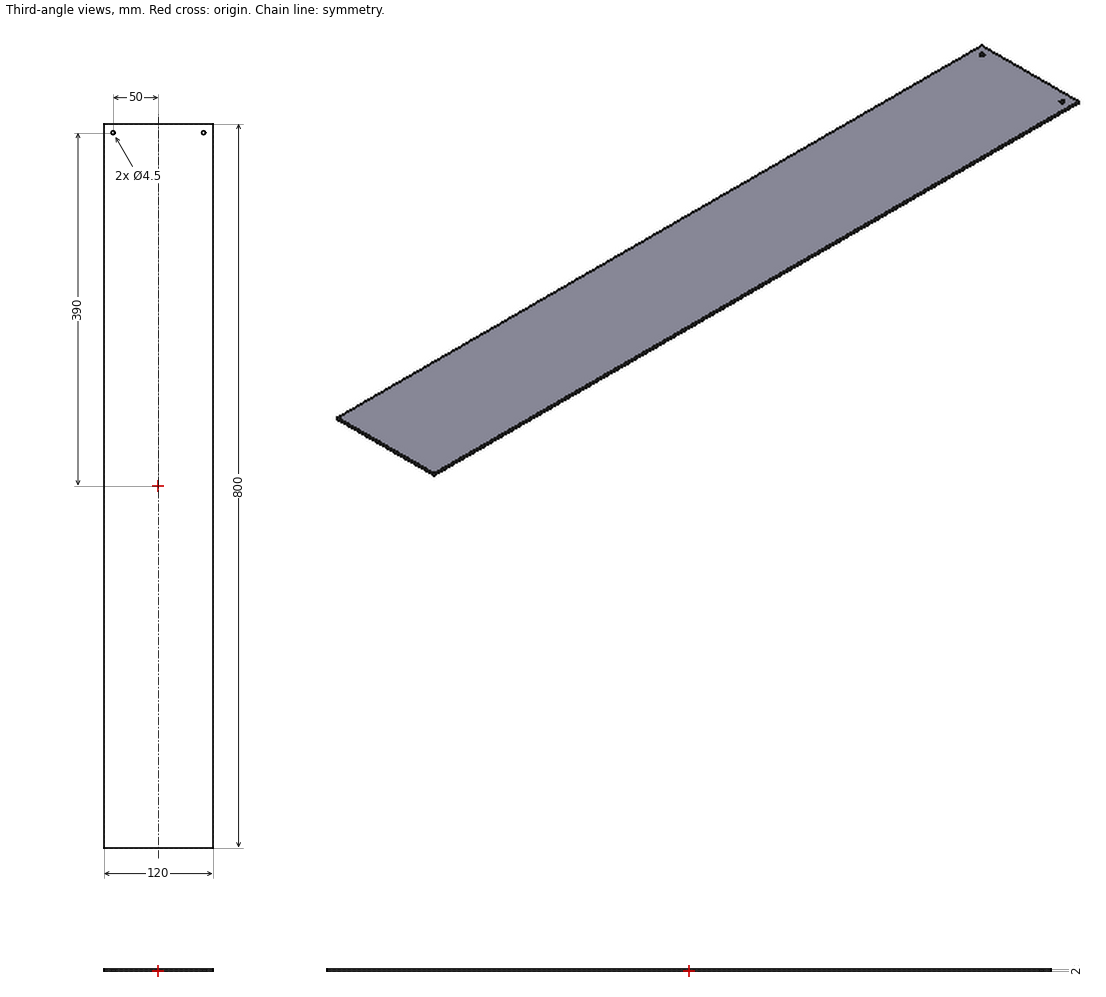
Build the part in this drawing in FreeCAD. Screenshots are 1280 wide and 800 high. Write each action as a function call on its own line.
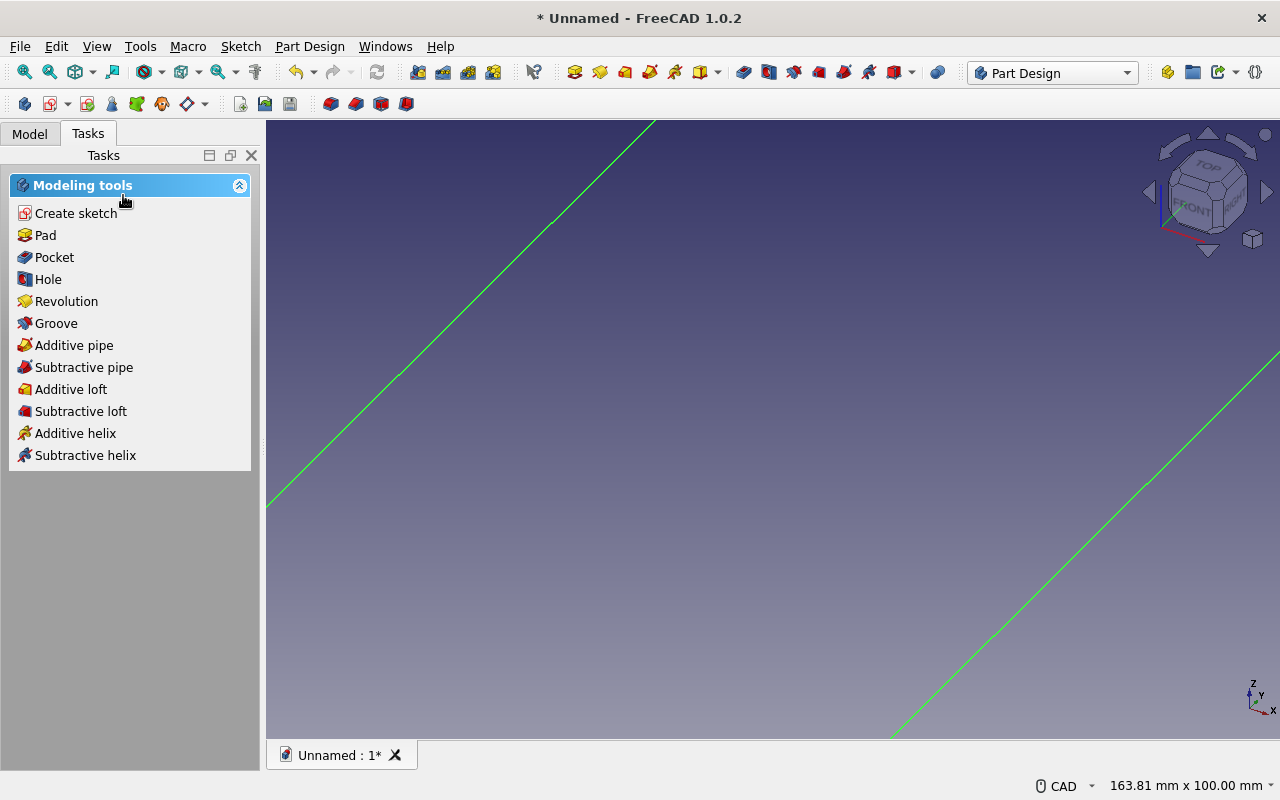
click(575, 72)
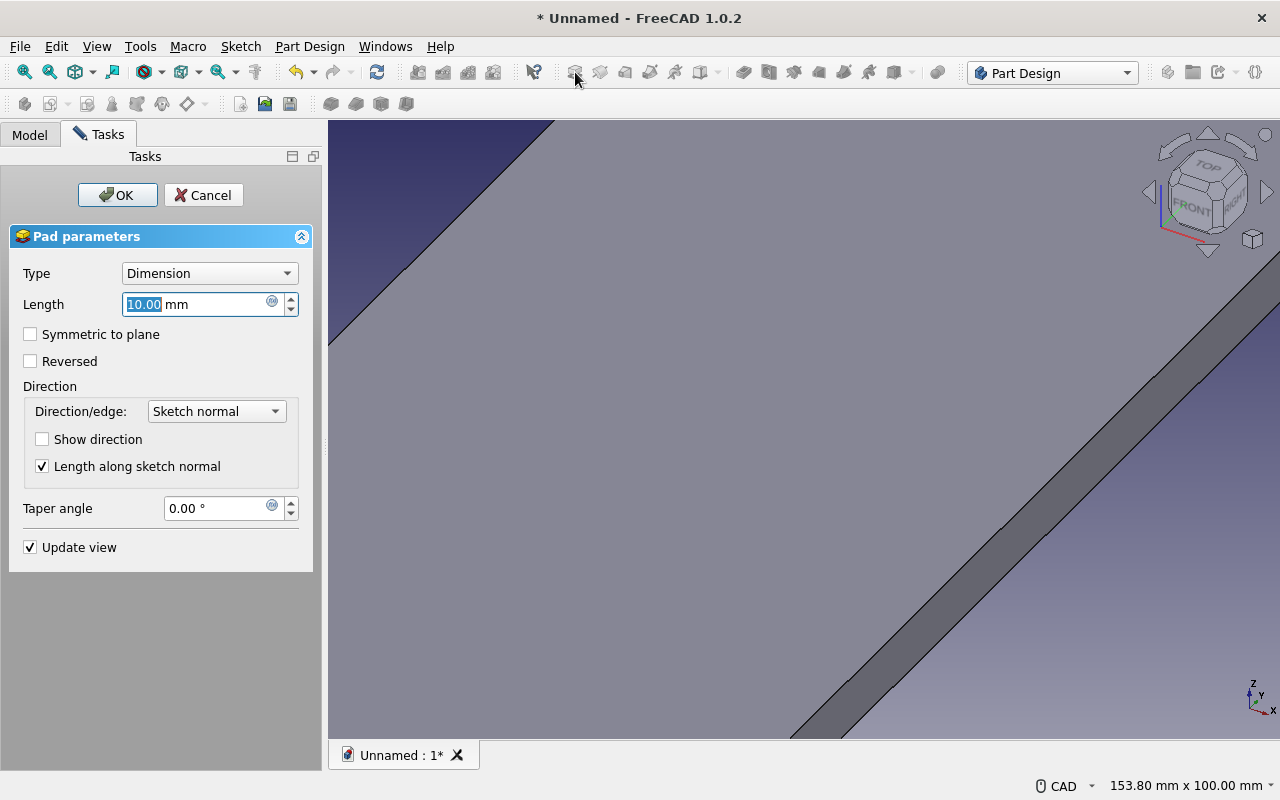
text(2)
key(Tab)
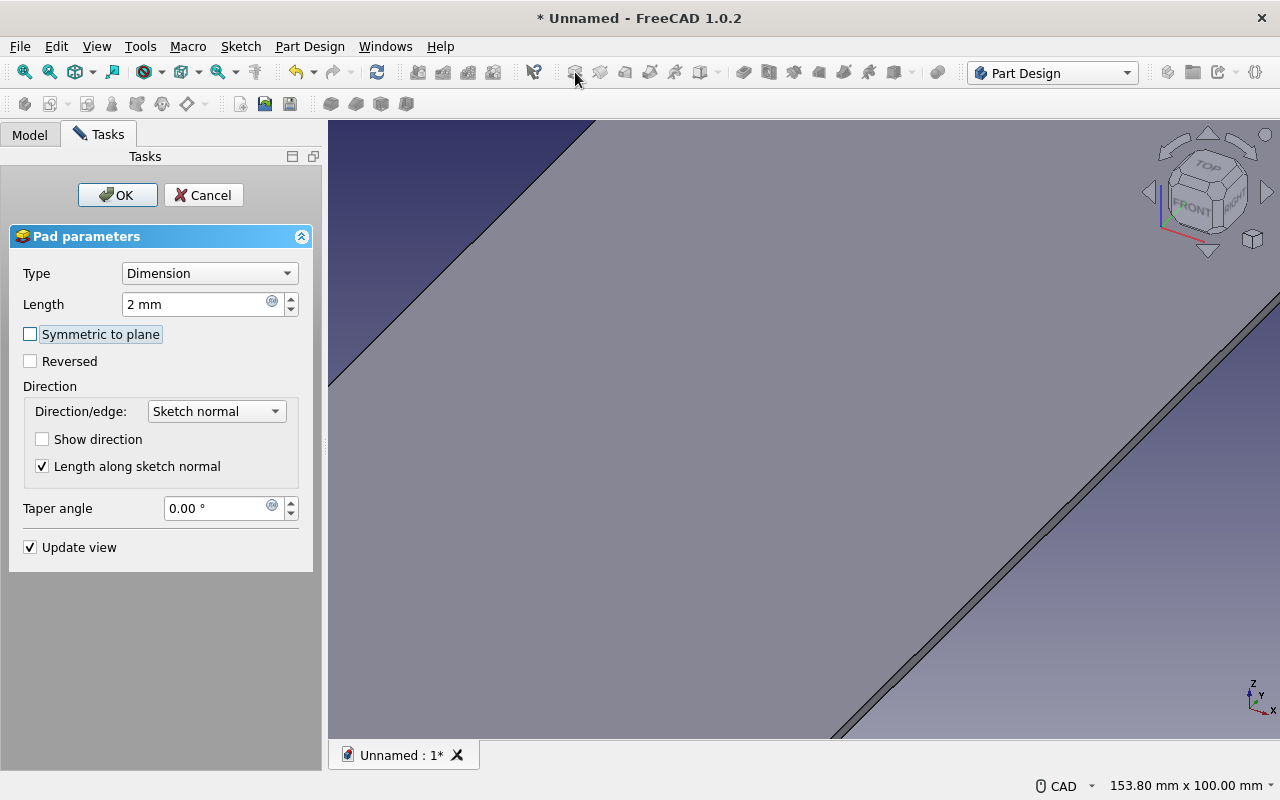
click(118, 195)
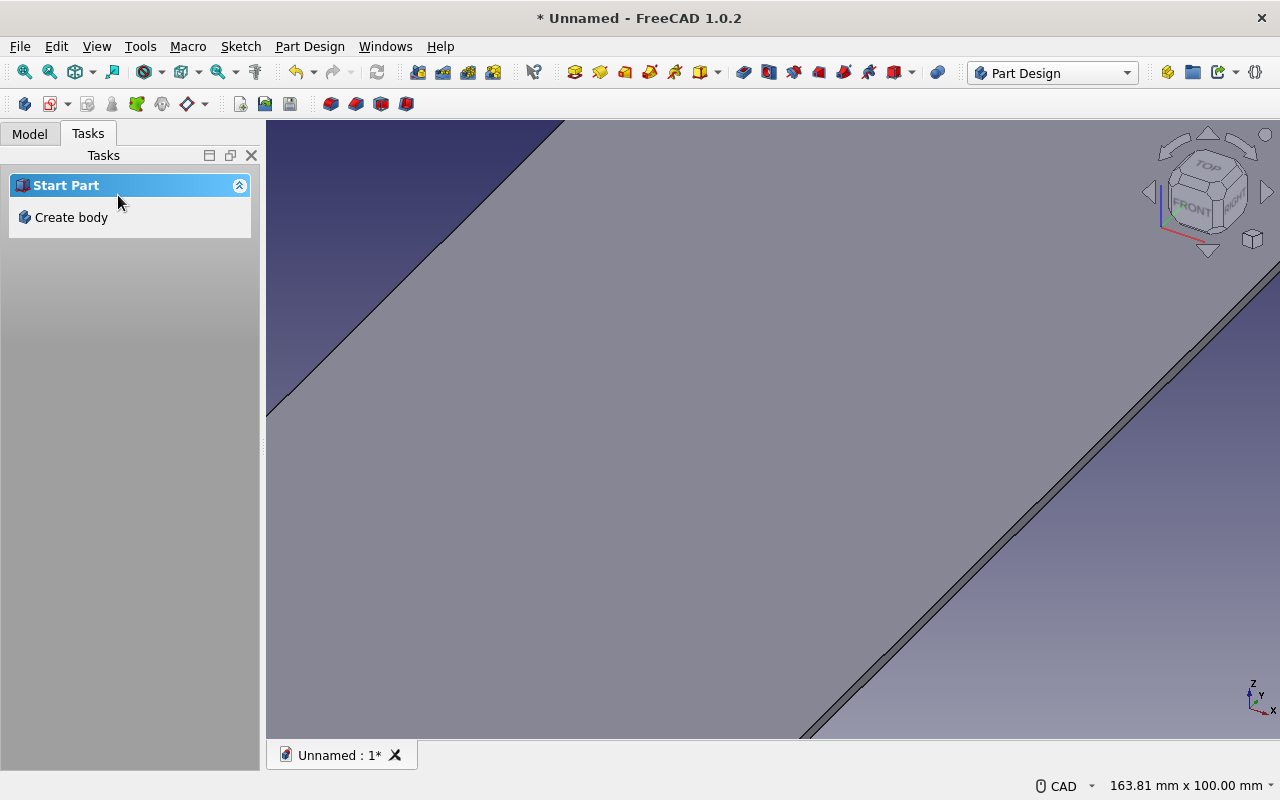
key(v)
key(f)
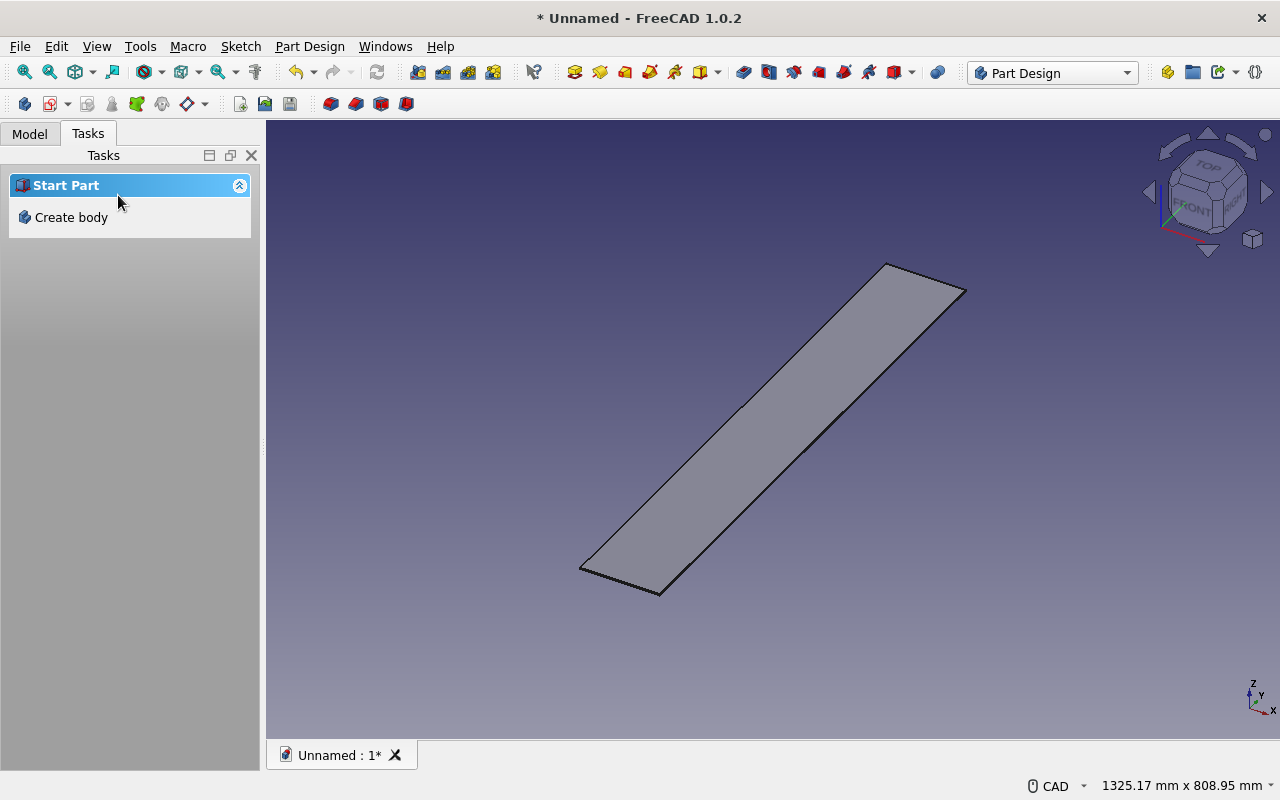
click(860, 341)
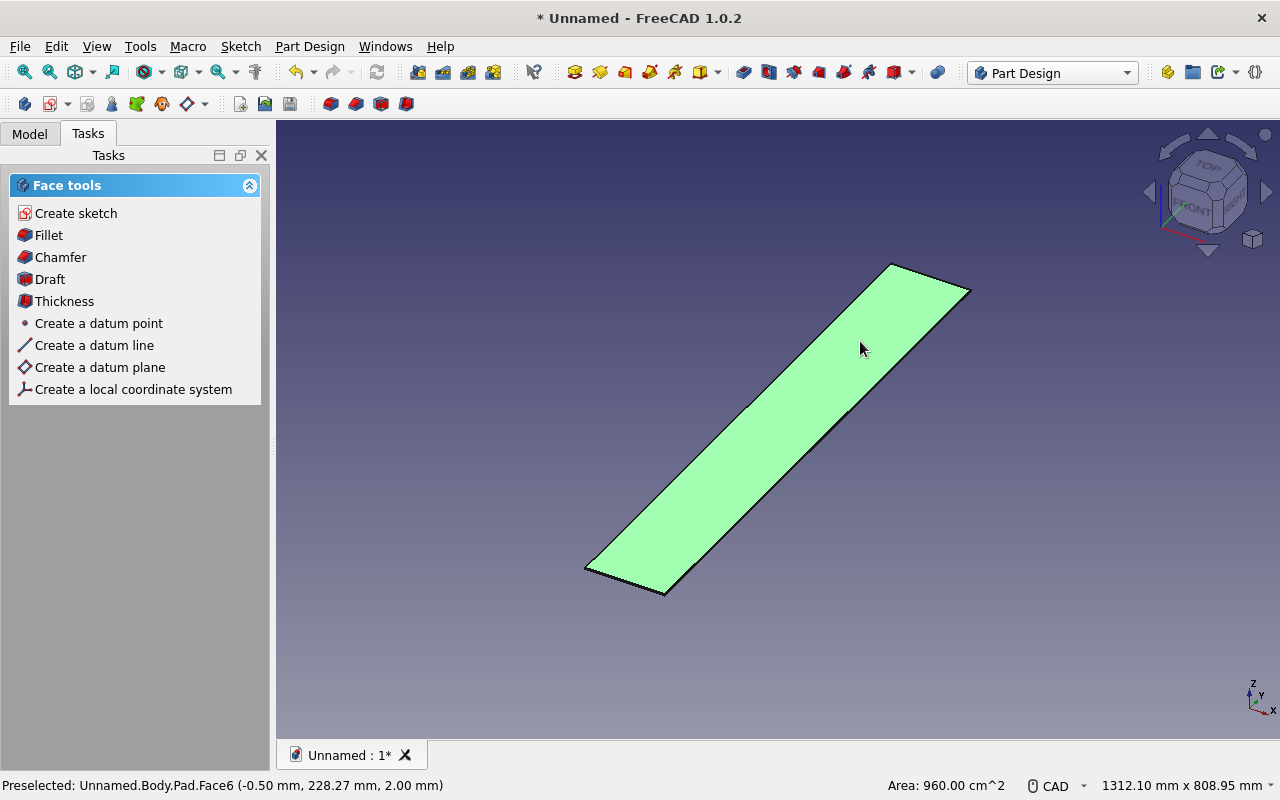
click(50, 104)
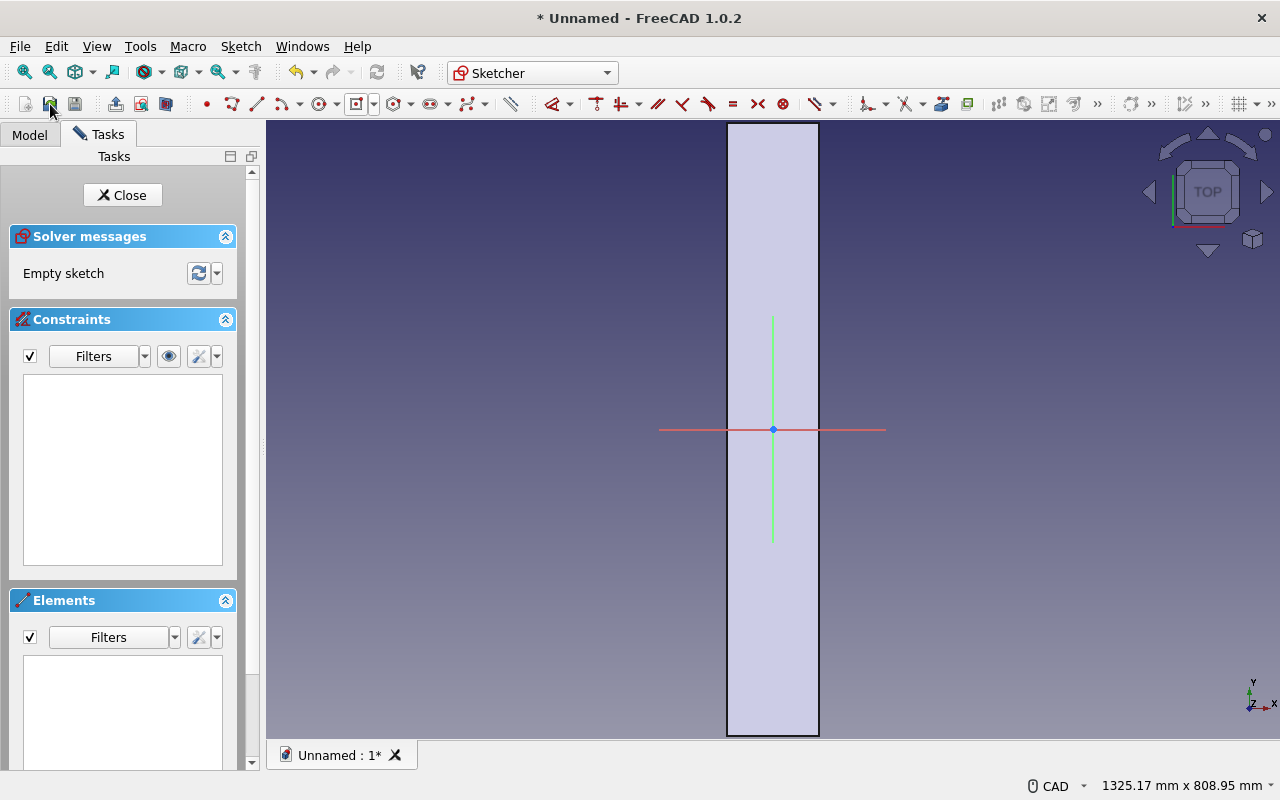
scroll(704, 430, down, 5)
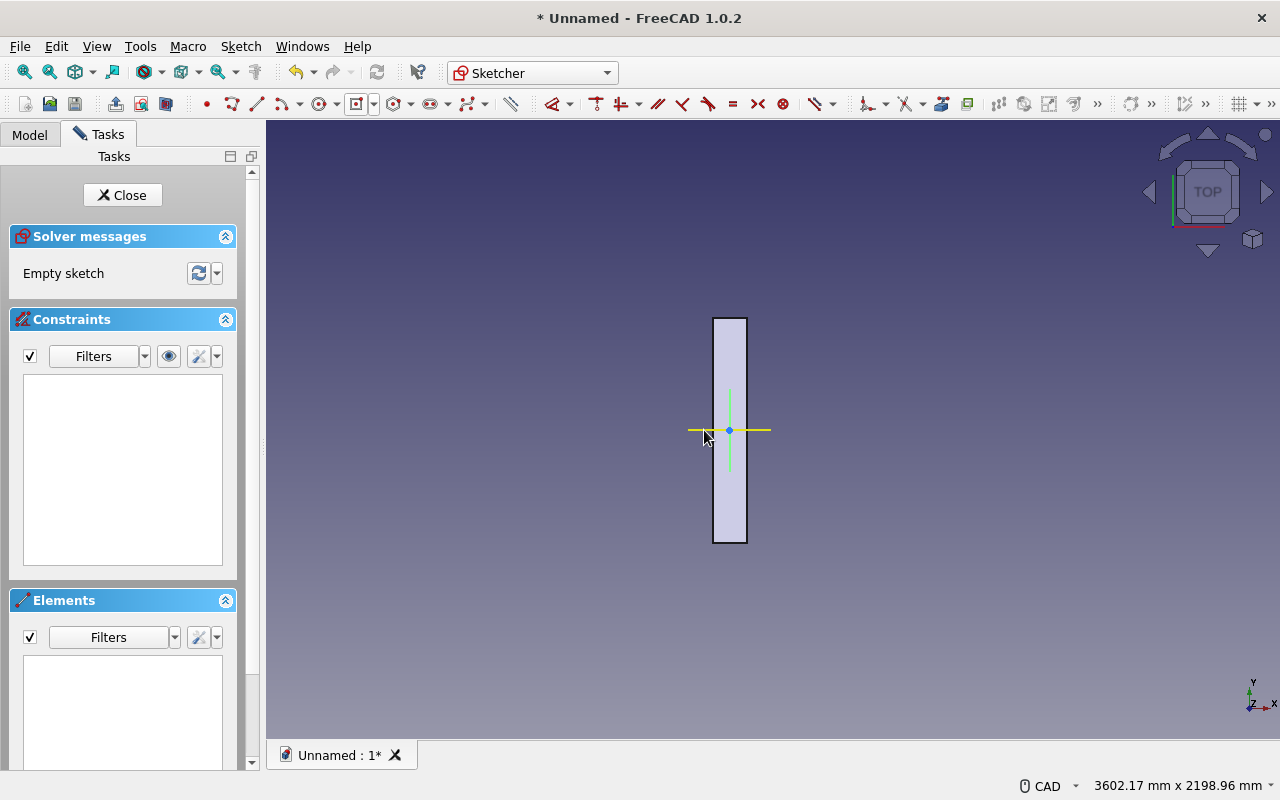
scroll(731, 315, up, 15)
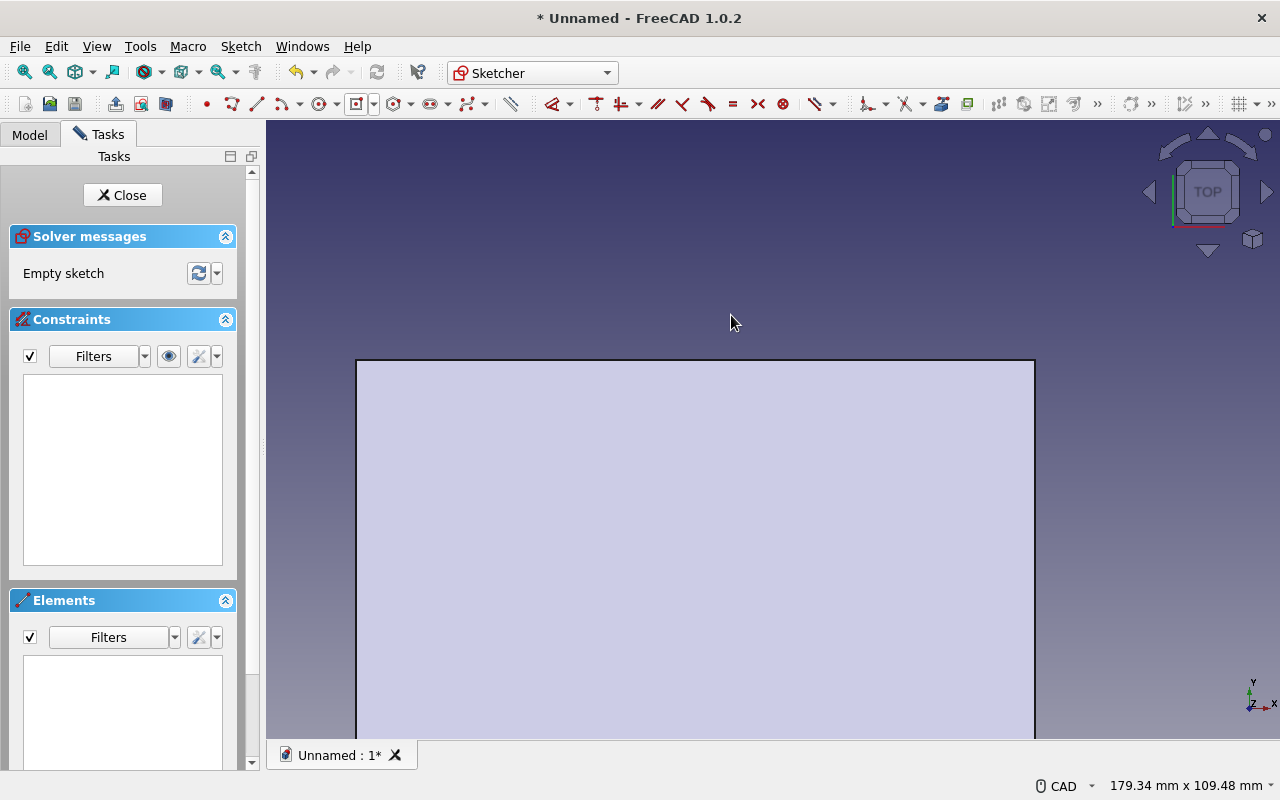
key(g)
key(c)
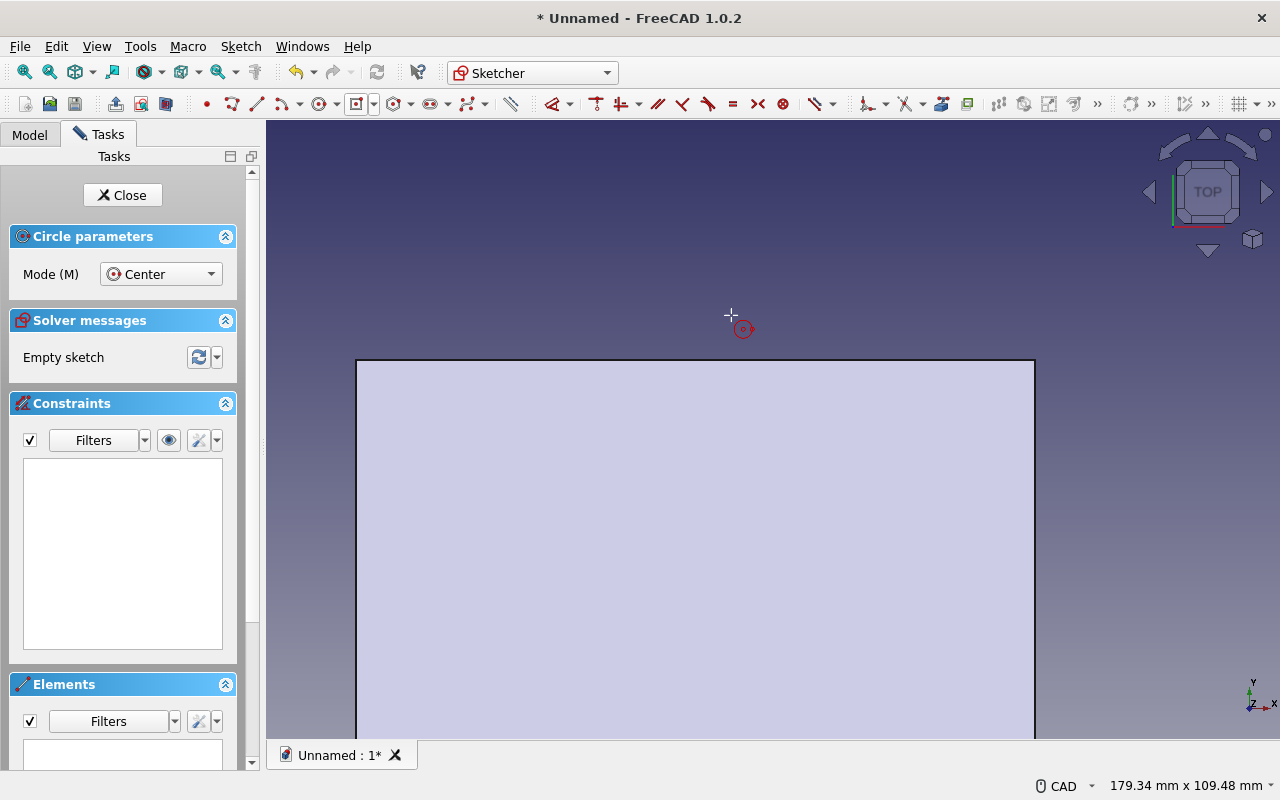
scroll(413, 416, up, 3)